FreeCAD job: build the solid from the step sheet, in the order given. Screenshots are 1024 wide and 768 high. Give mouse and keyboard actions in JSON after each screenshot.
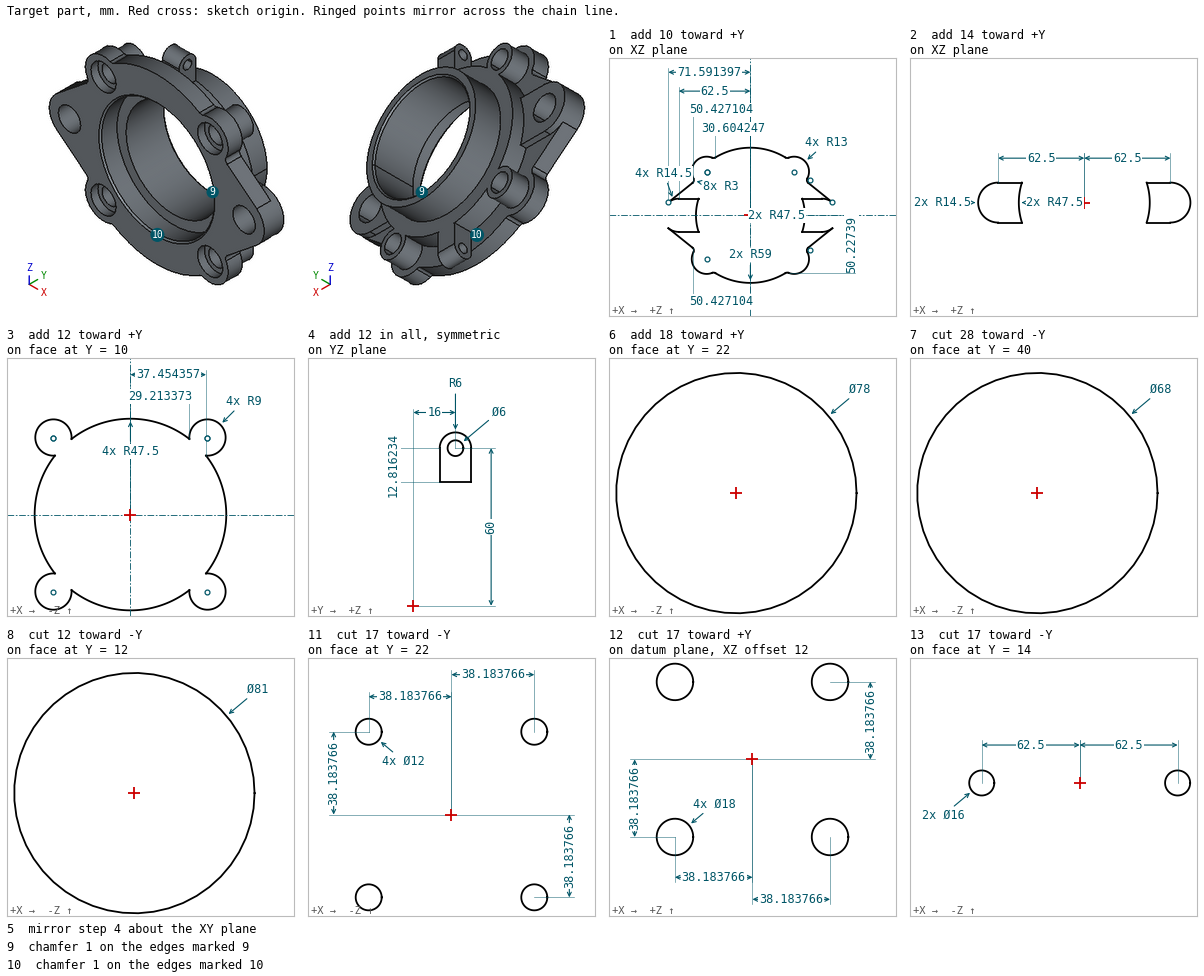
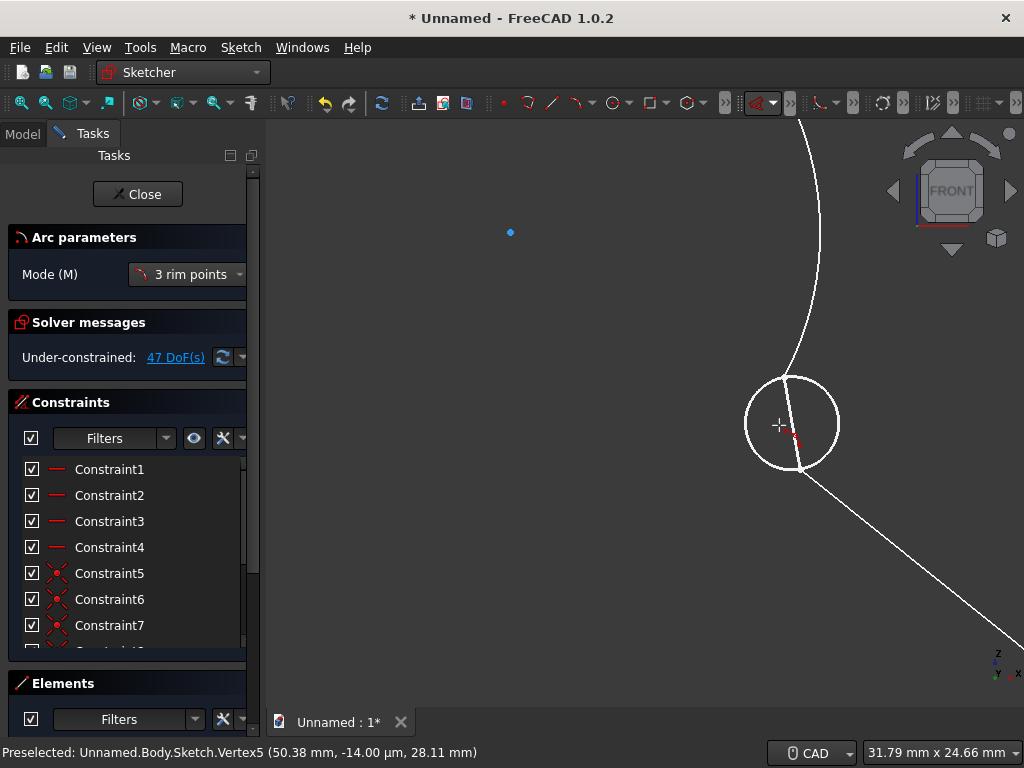
{"action": "left_click", "coordinate": [776, 423]}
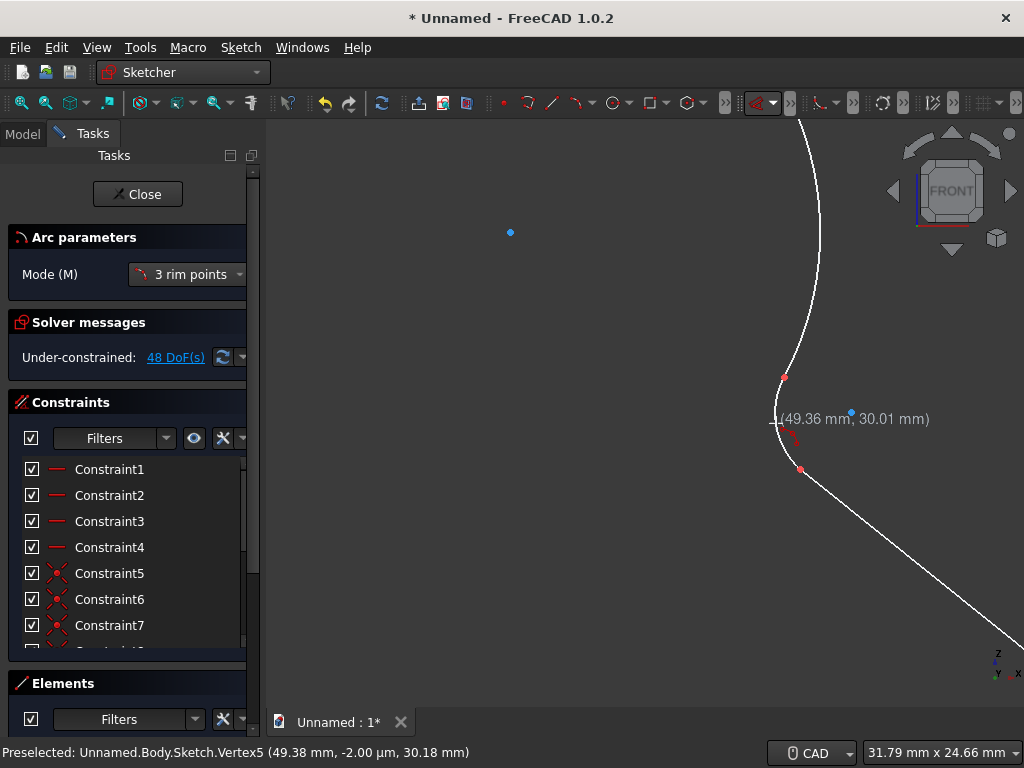
{"action": "scroll", "coordinate": [698, 322], "scroll_direction": "down", "scroll_amount": 11}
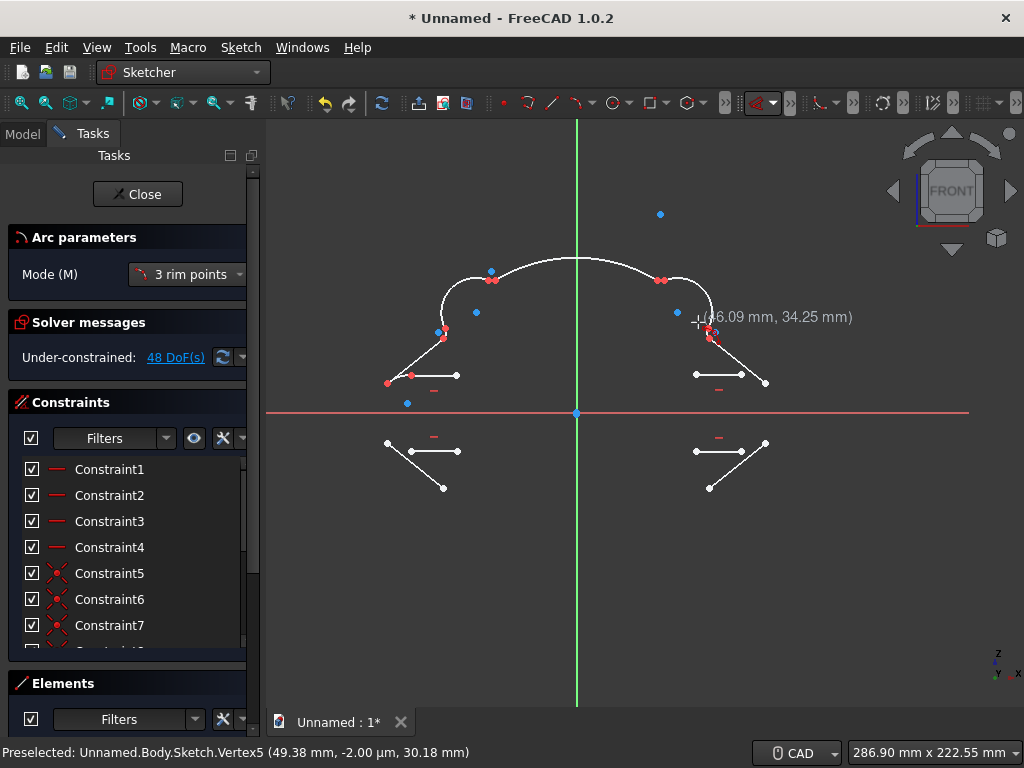
{"action": "left_click", "coordinate": [766, 384]}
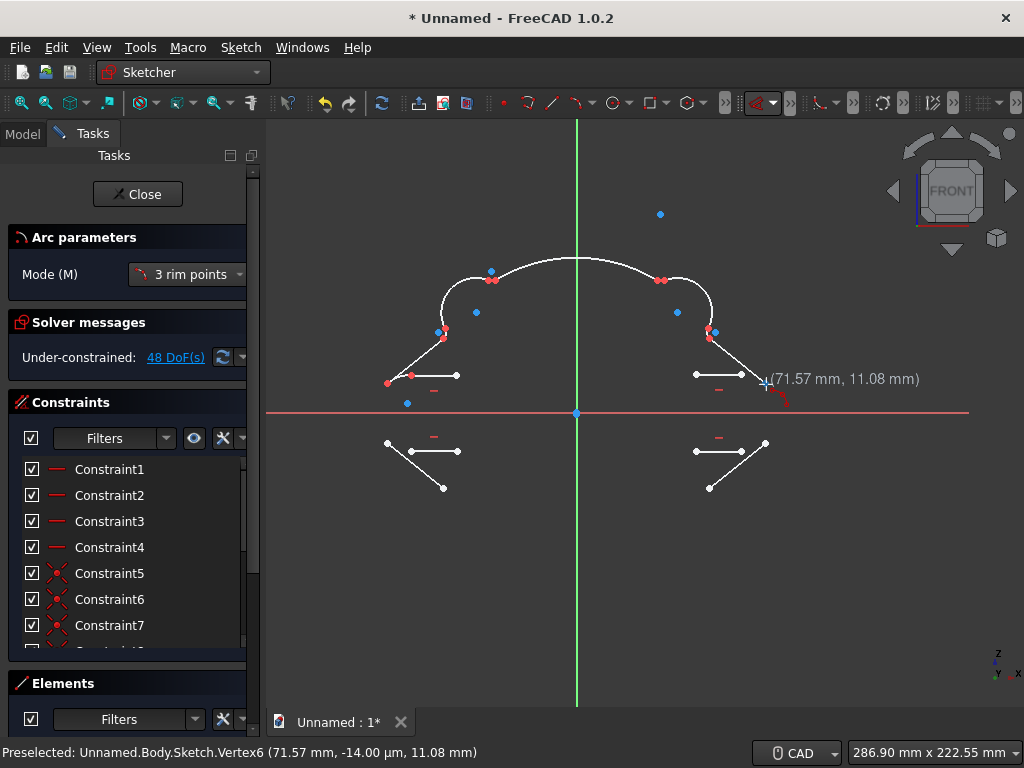
{"action": "scroll", "coordinate": [742, 375], "scroll_direction": "up", "scroll_amount": 4}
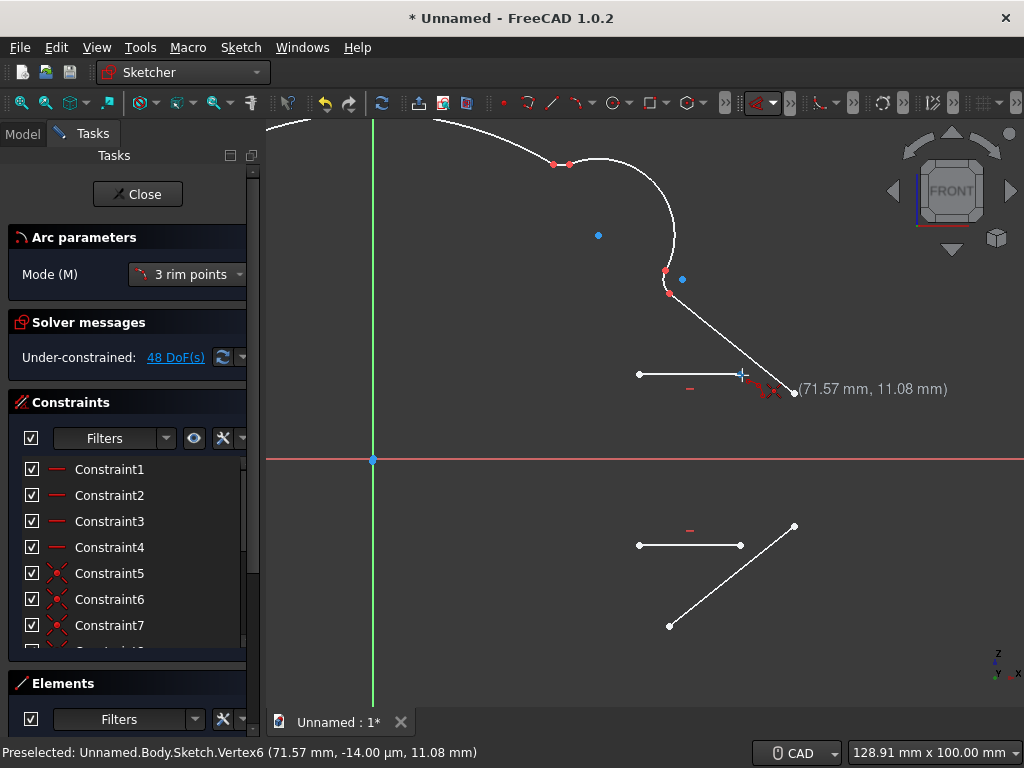
{"action": "left_click", "coordinate": [741, 374]}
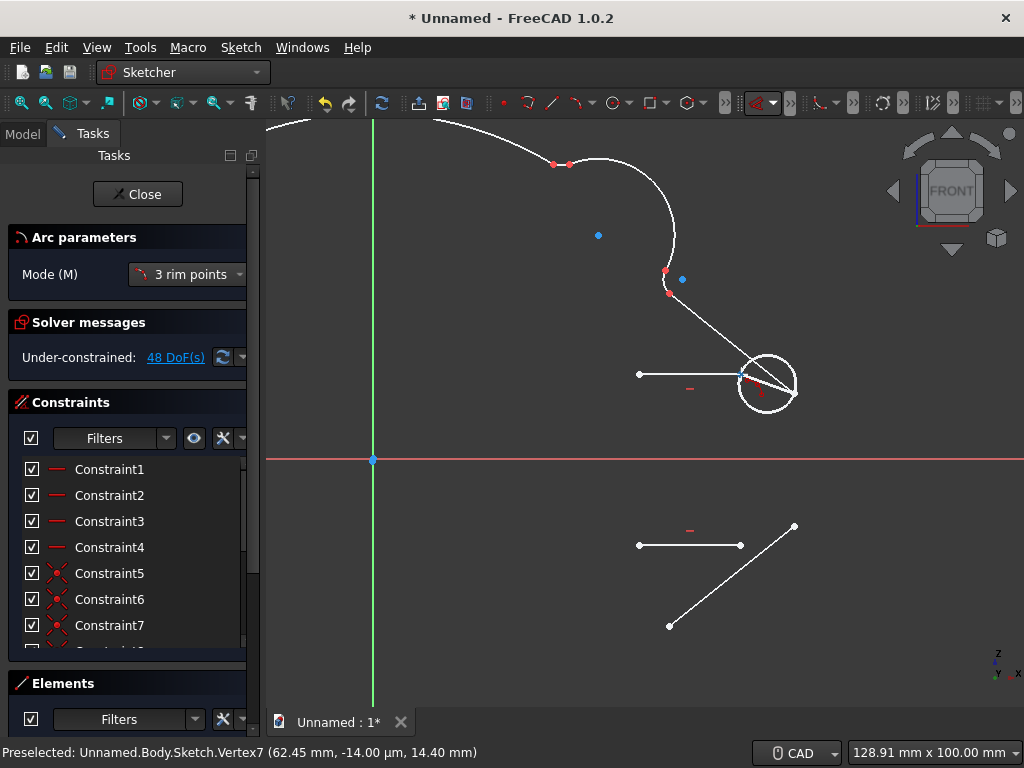
{"action": "scroll", "coordinate": [769, 378], "scroll_direction": "up", "scroll_amount": 6}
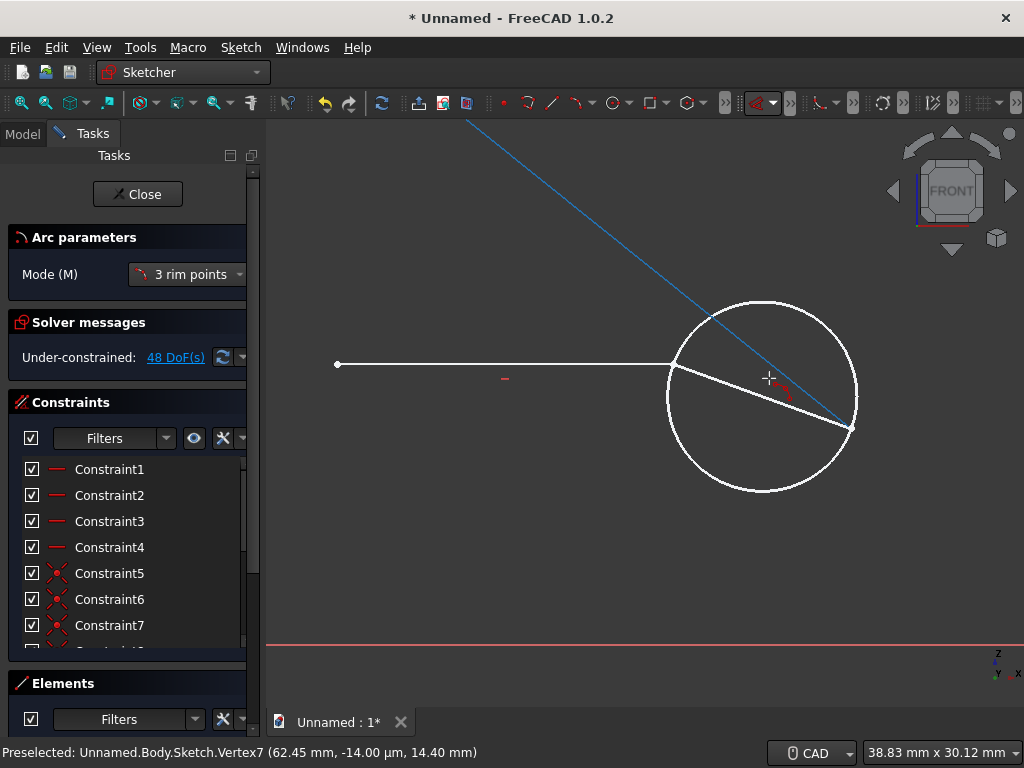
{"action": "left_click", "coordinate": [768, 378]}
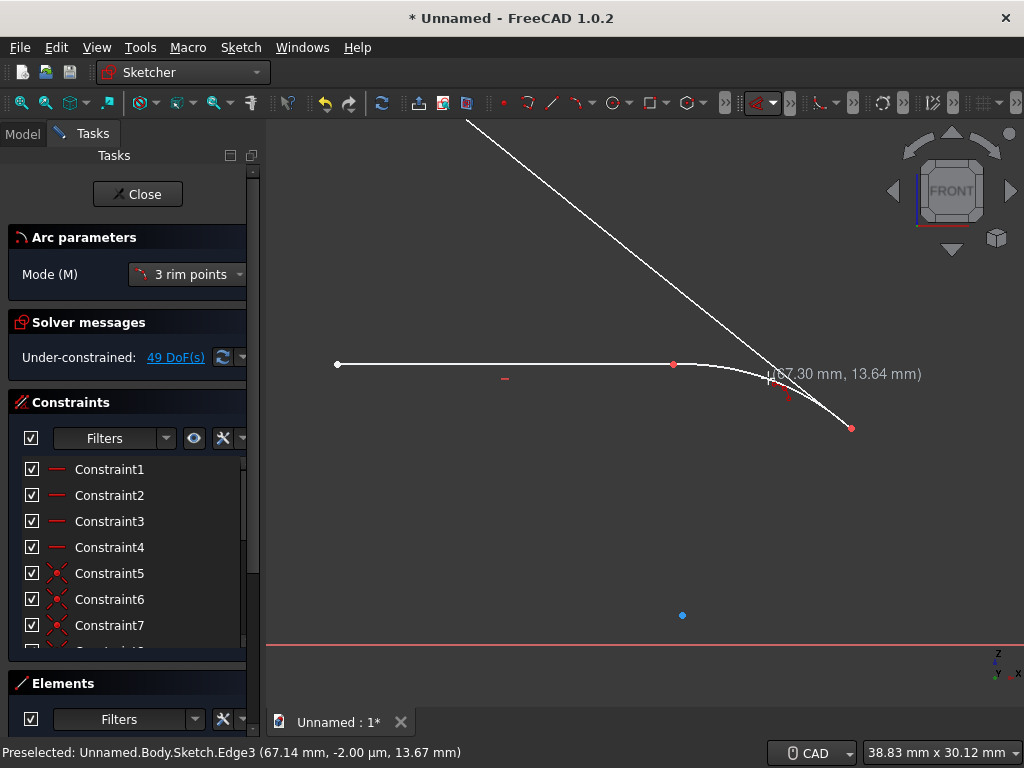
{"action": "scroll", "coordinate": [752, 377], "scroll_direction": "down", "scroll_amount": 10}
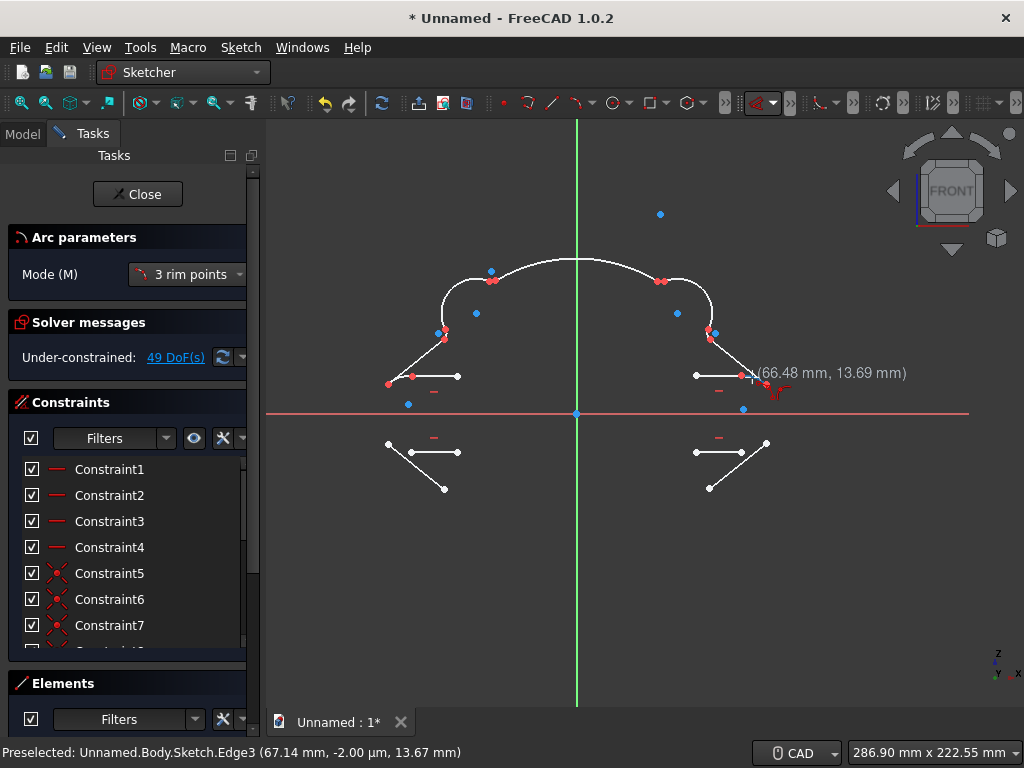
{"action": "left_click", "coordinate": [697, 376]}
{"action": "left_click", "coordinate": [697, 452]}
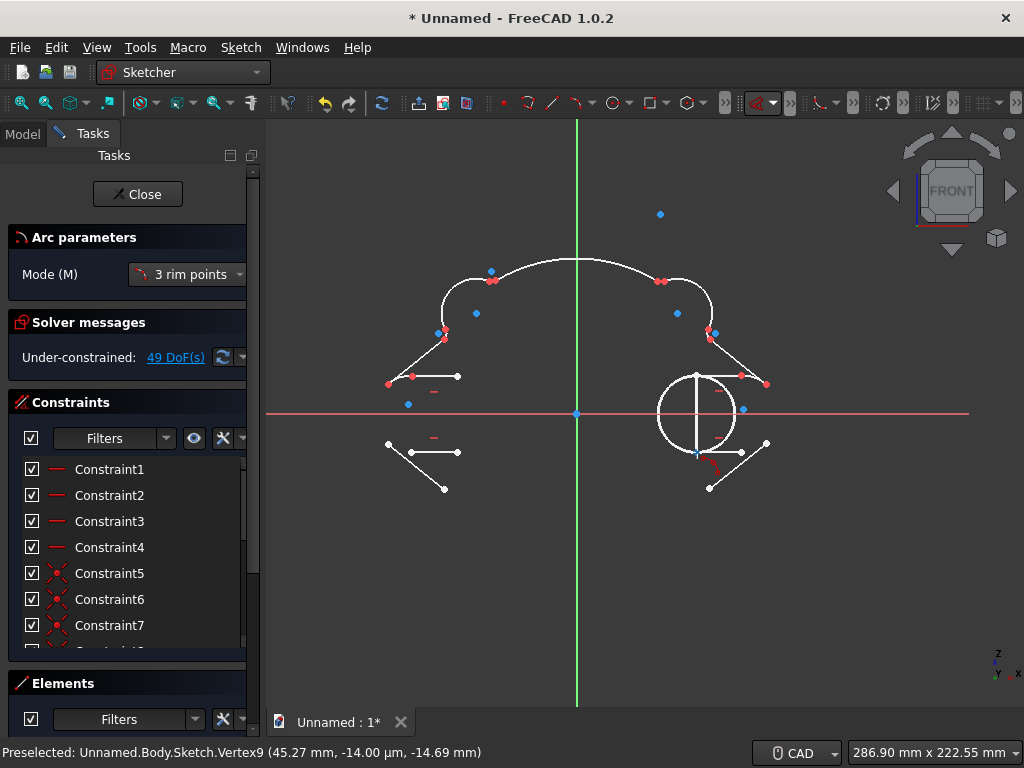
{"action": "scroll", "coordinate": [702, 421], "scroll_direction": "up", "scroll_amount": 6}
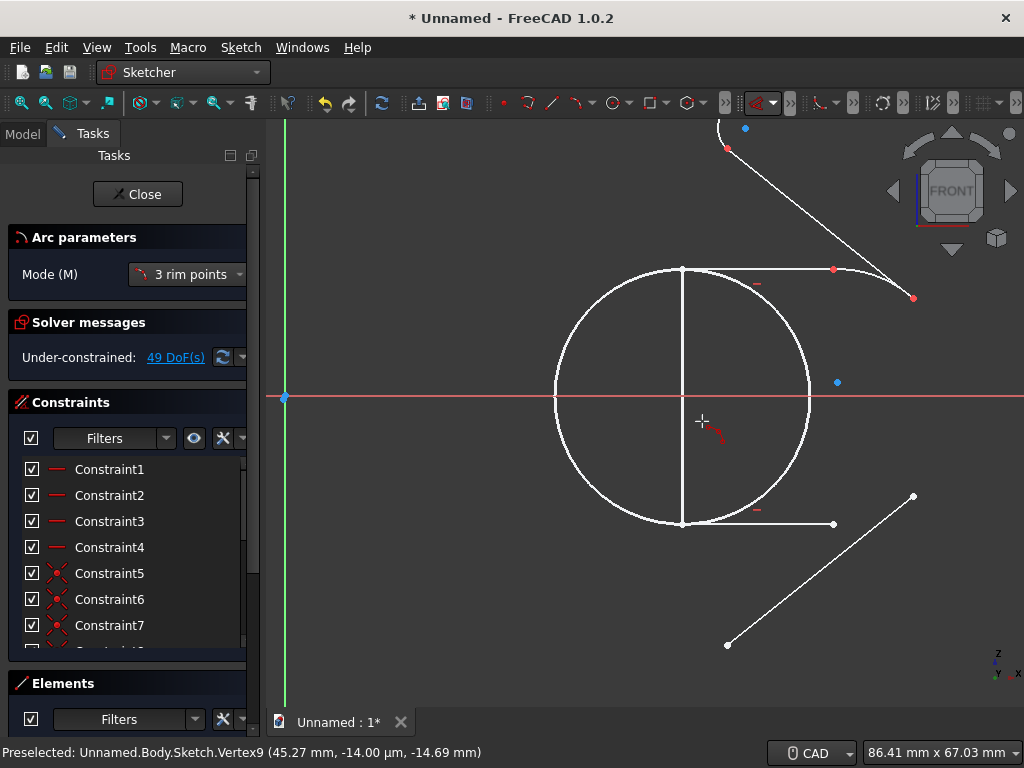
{"action": "left_click", "coordinate": [701, 421]}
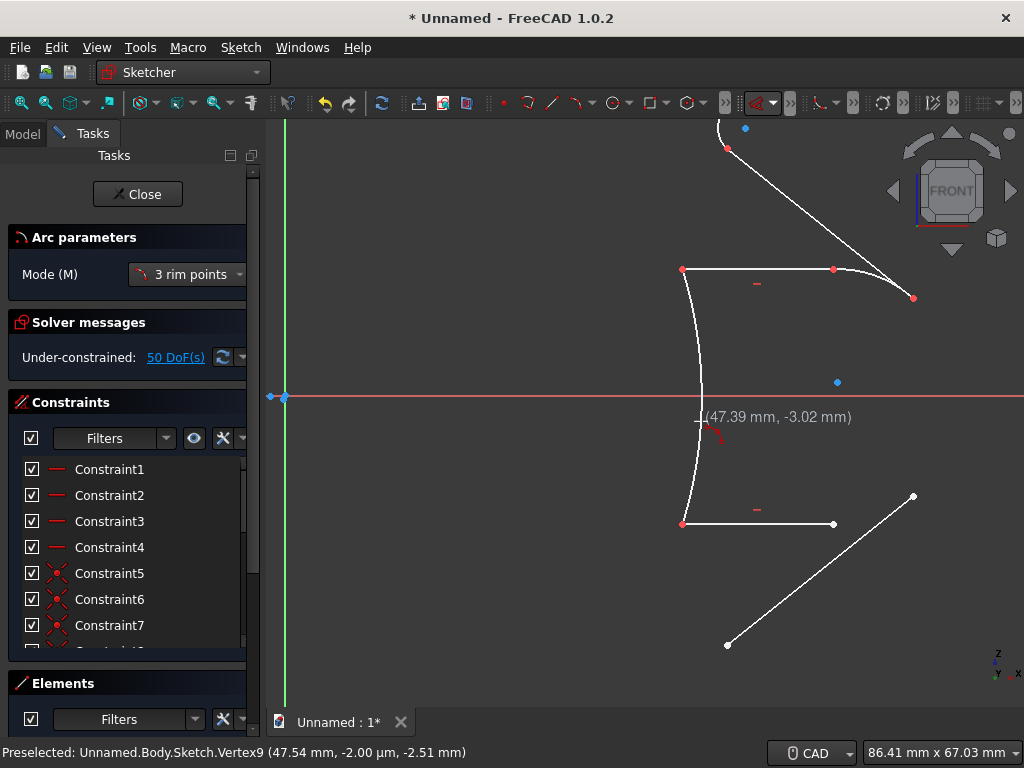
{"action": "left_click", "coordinate": [833, 524]}